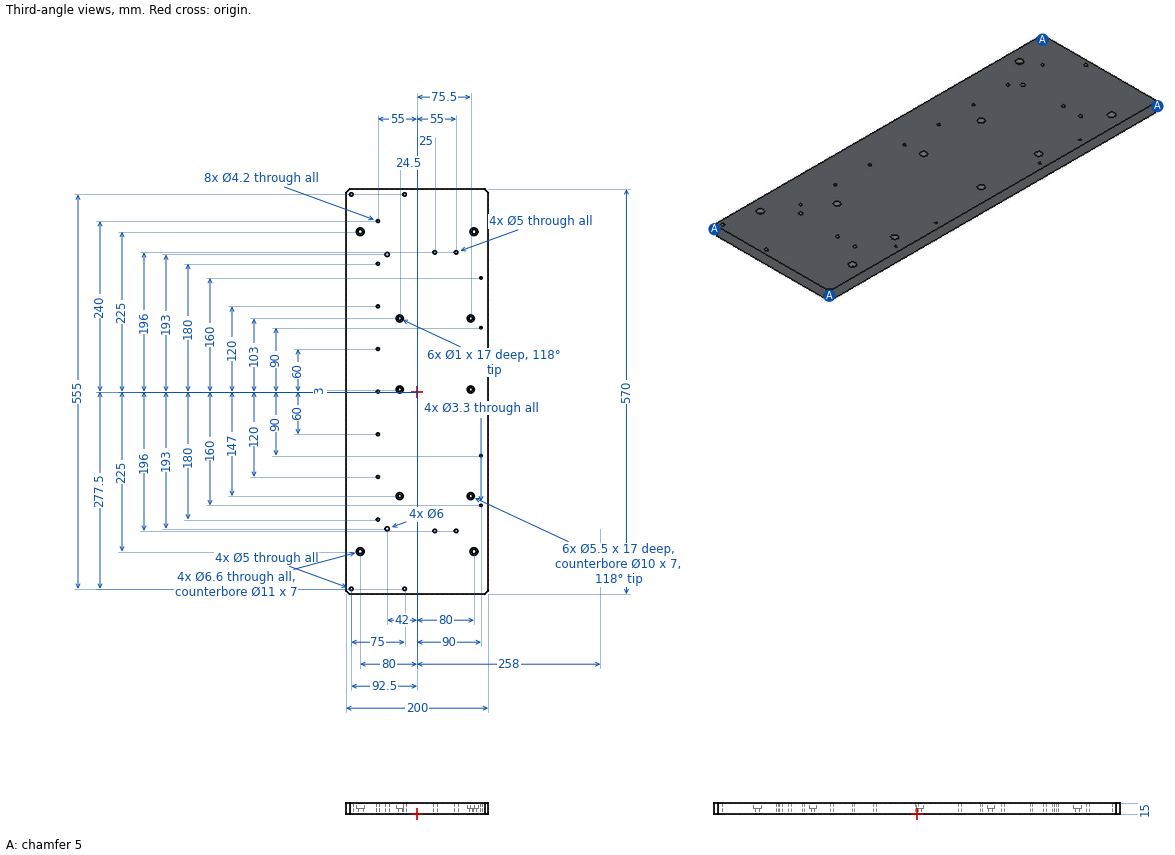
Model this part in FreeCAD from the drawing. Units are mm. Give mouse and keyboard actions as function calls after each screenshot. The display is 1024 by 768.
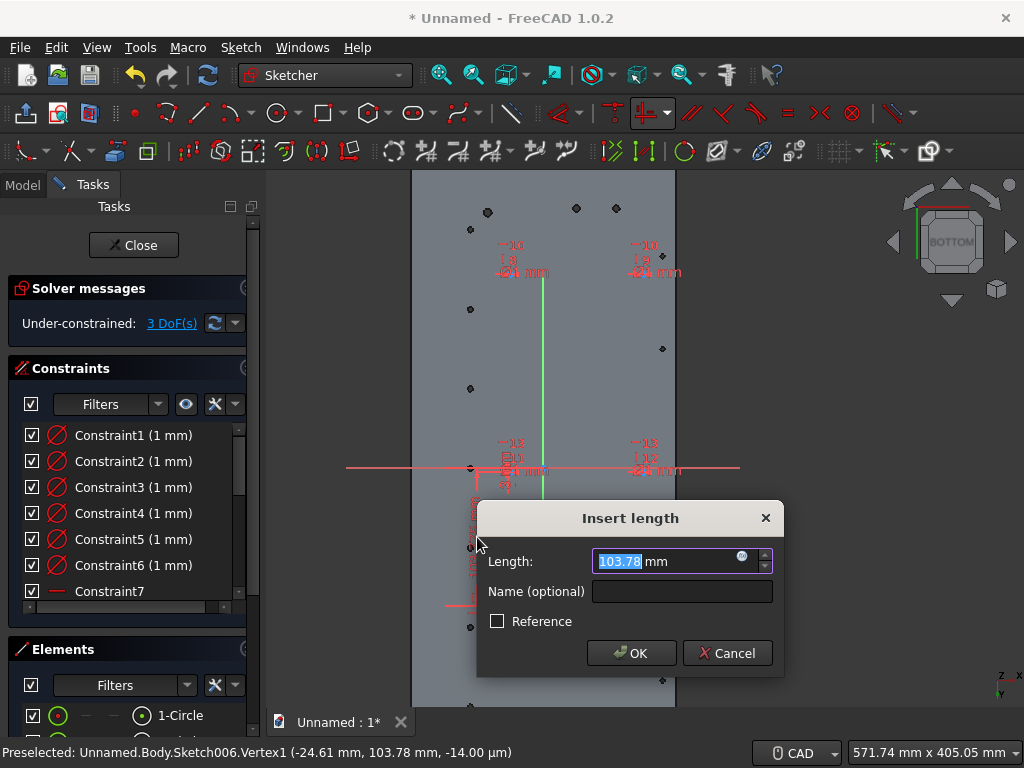
text(103)
key(Return)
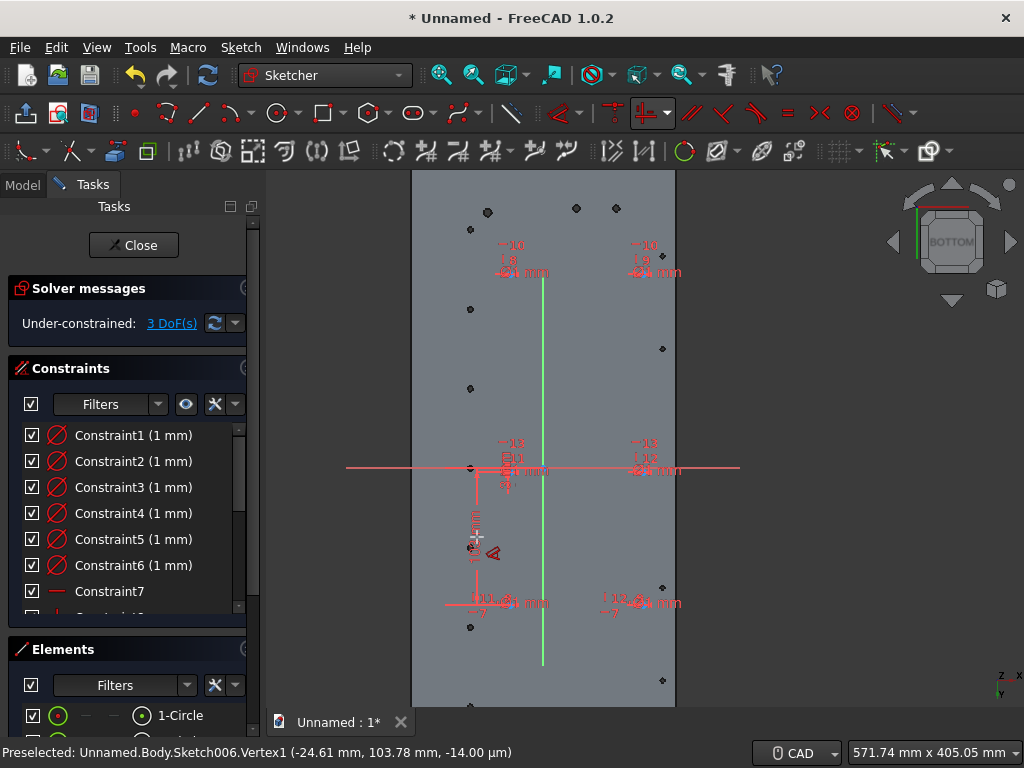
click(511, 274)
click(477, 371)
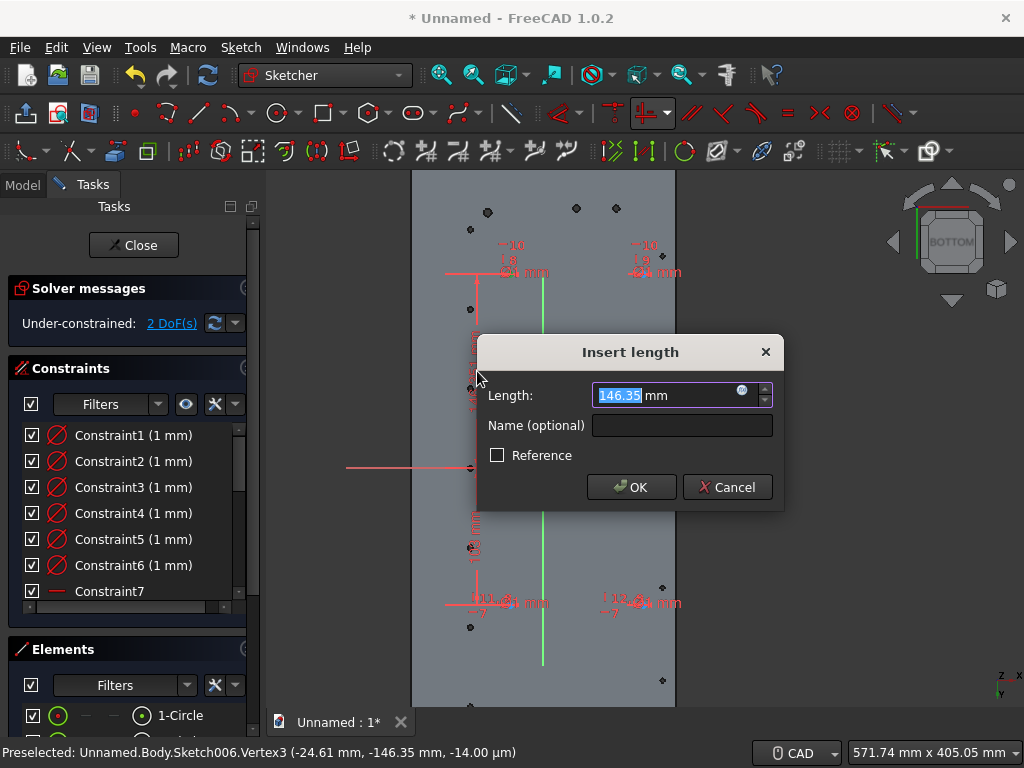
text(147)
key(Return)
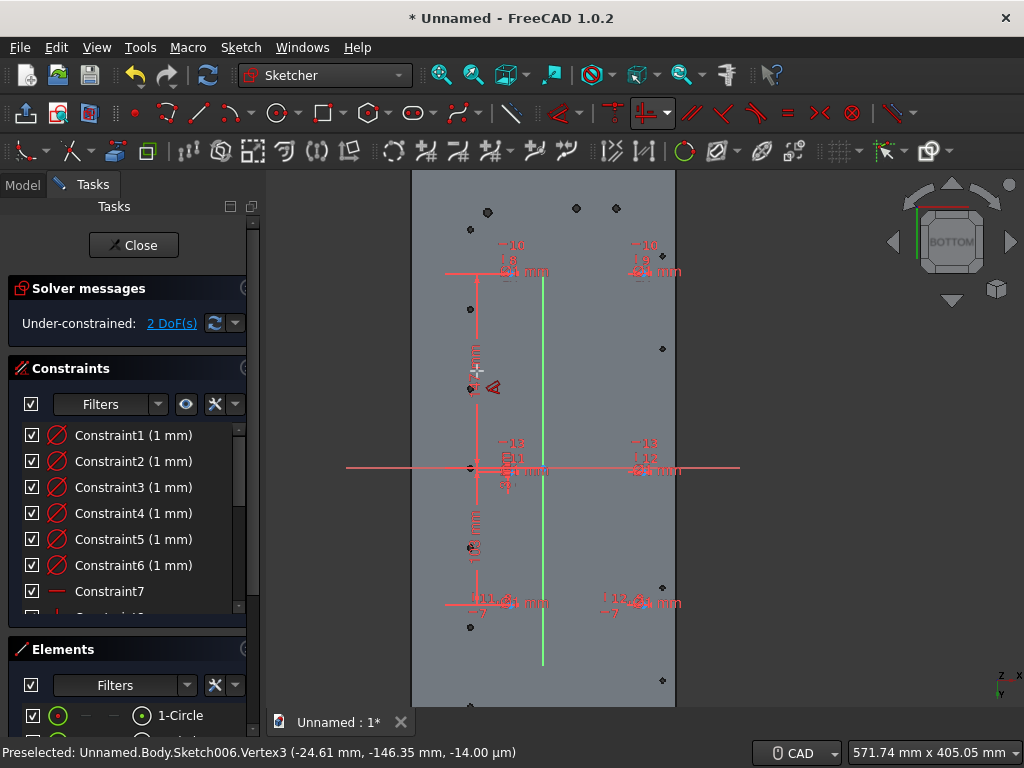
scroll(511, 605, up, 2)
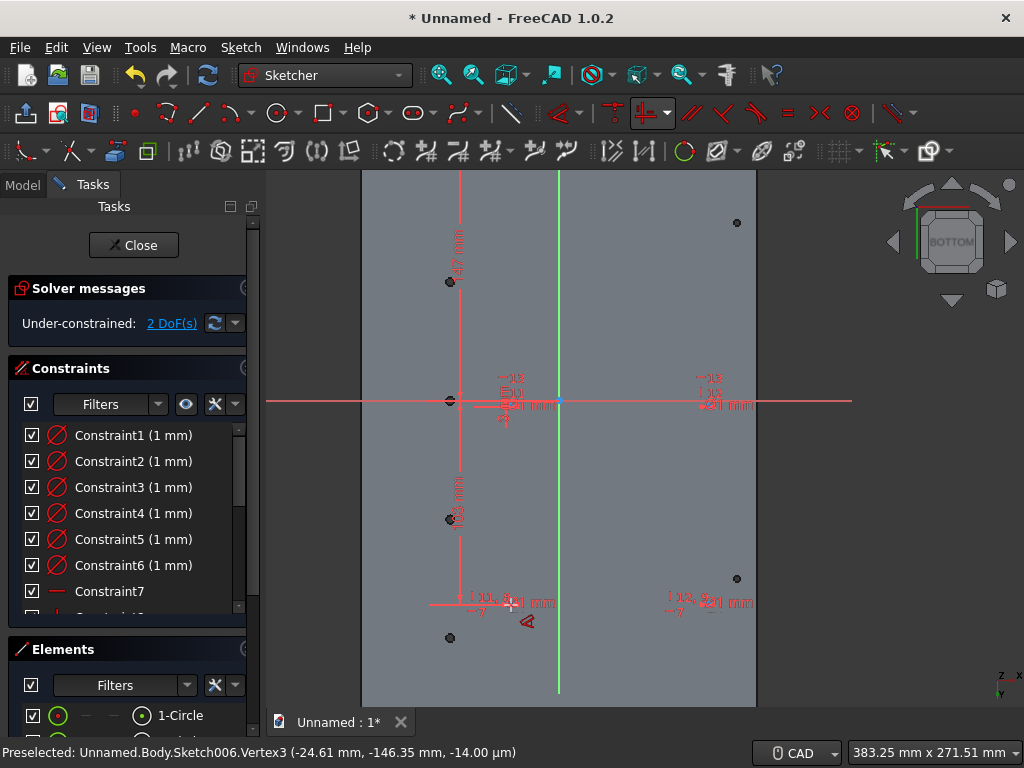
click(510, 605)
click(535, 639)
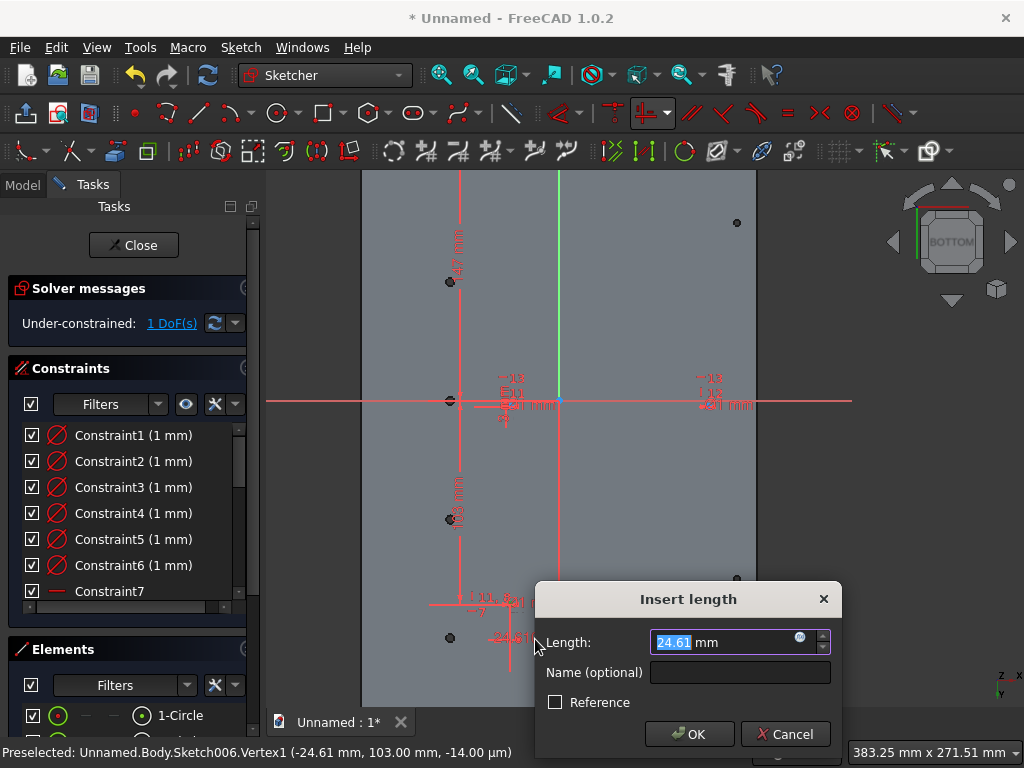
text(24.5)
key(Return)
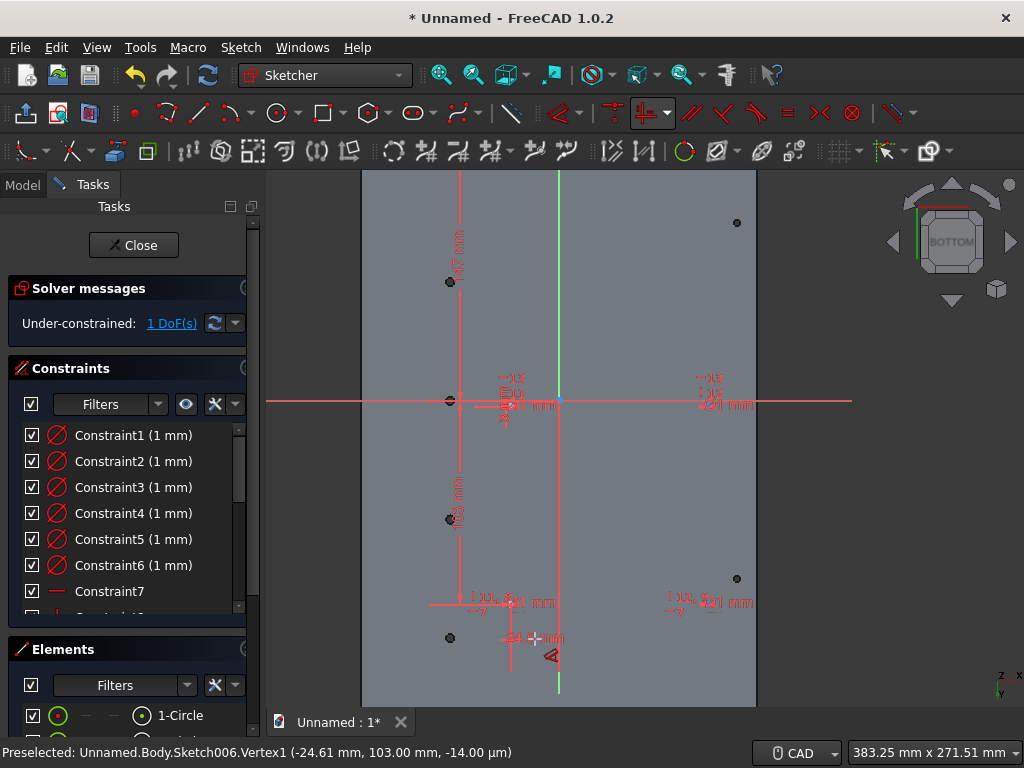
click(708, 605)
click(634, 639)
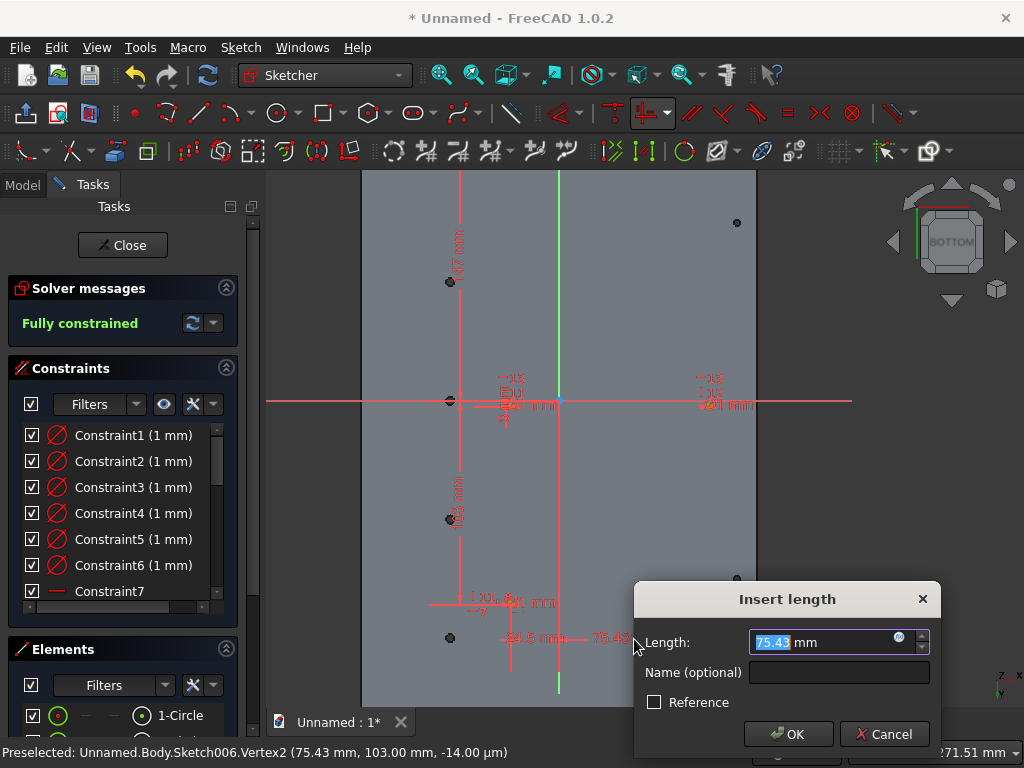
text(75.5)
key(Return)
key(Escape)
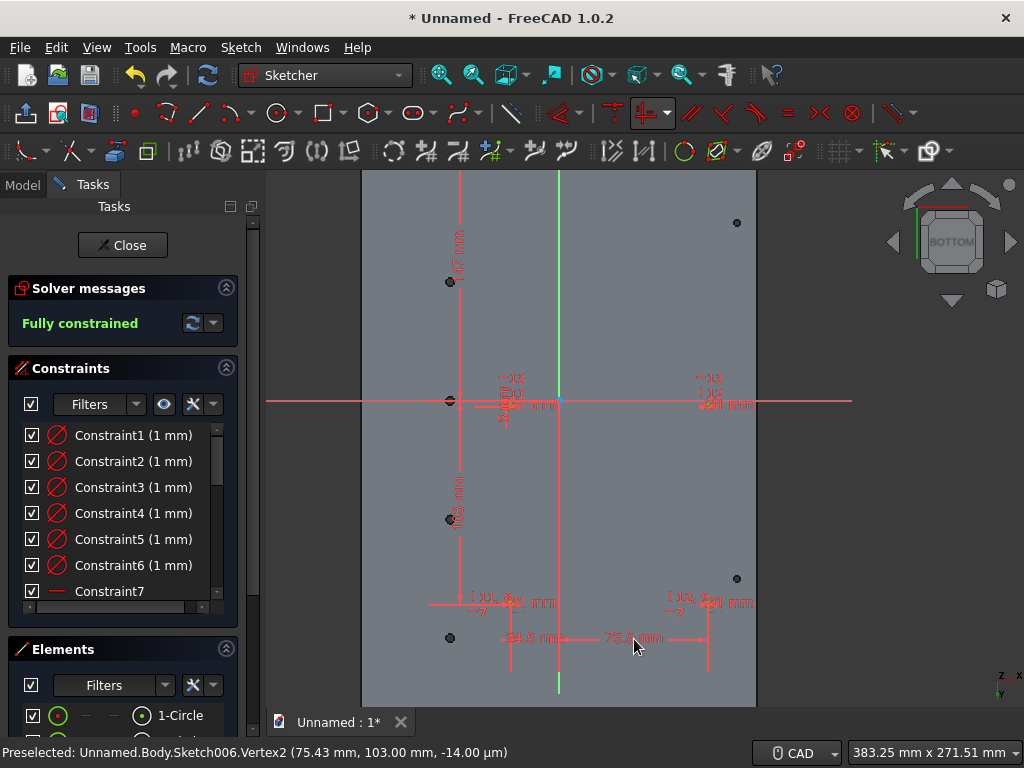
click(123, 245)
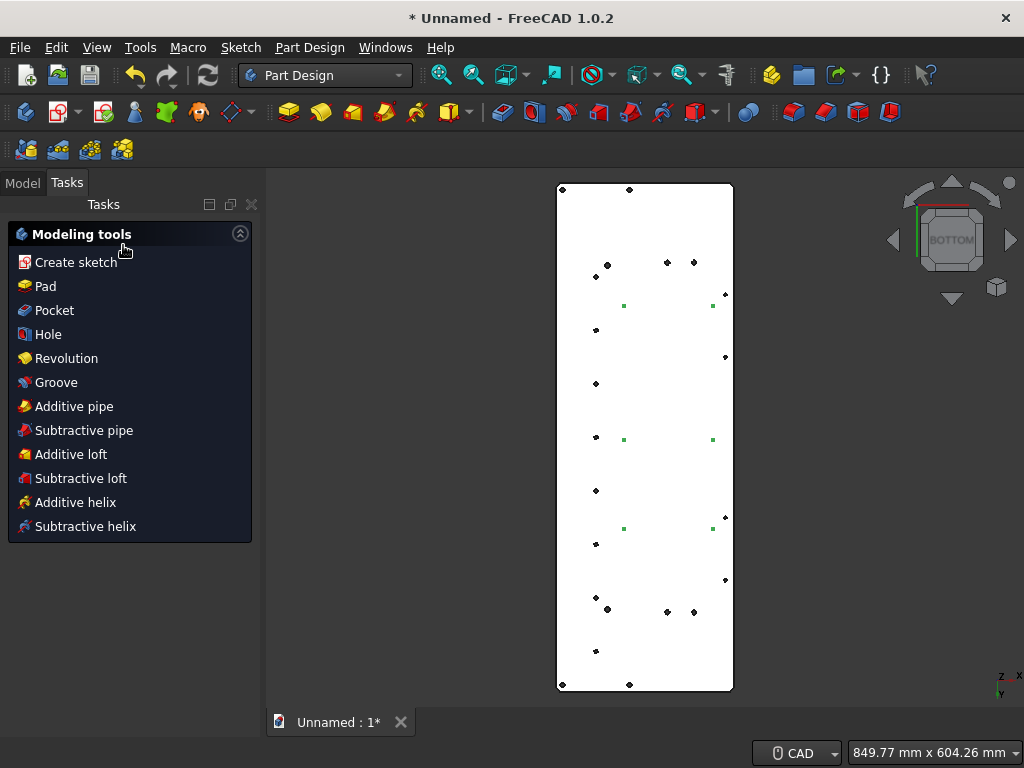
click(536, 112)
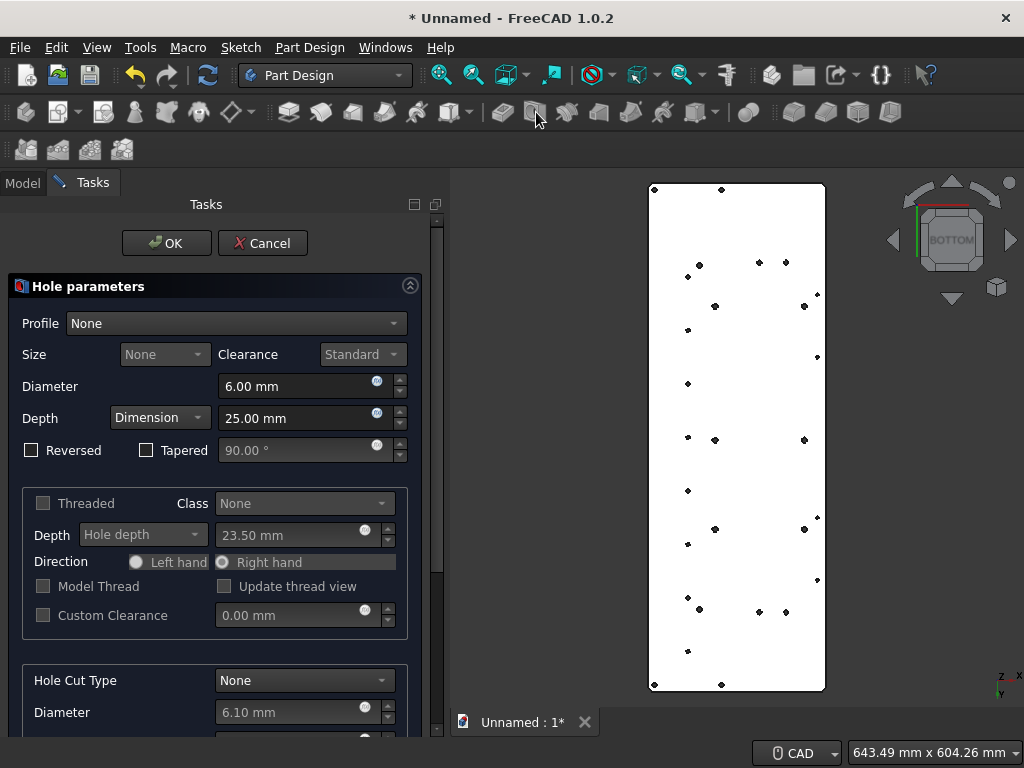
triple_click(305, 386)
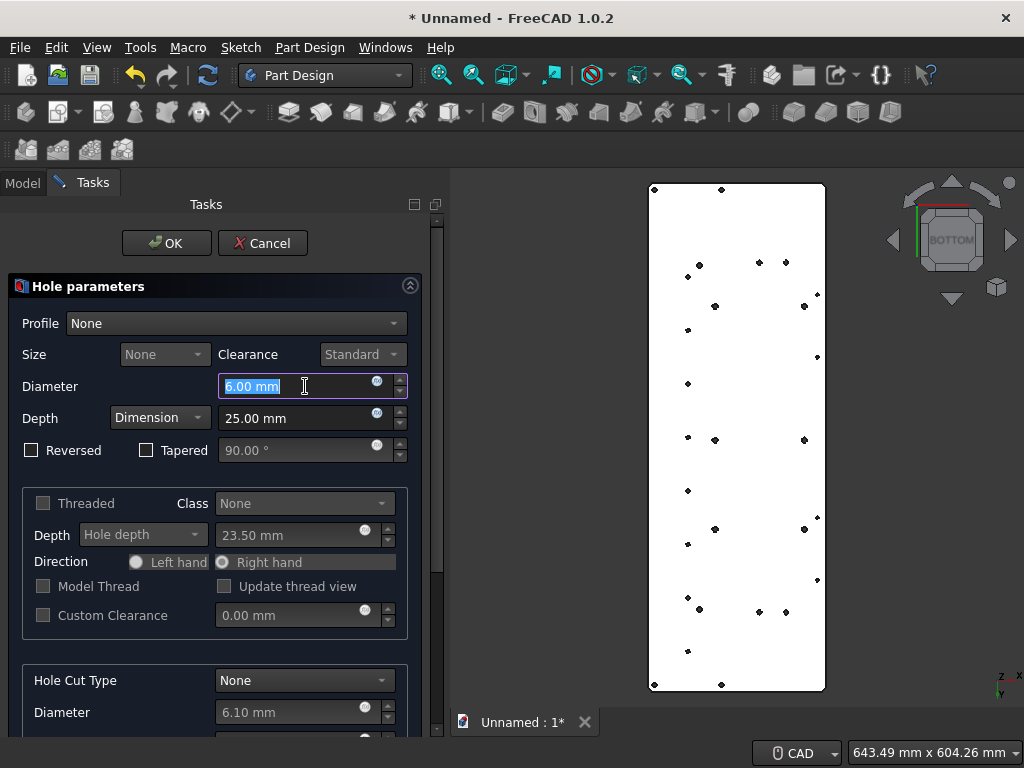
text(1)
key(Tab)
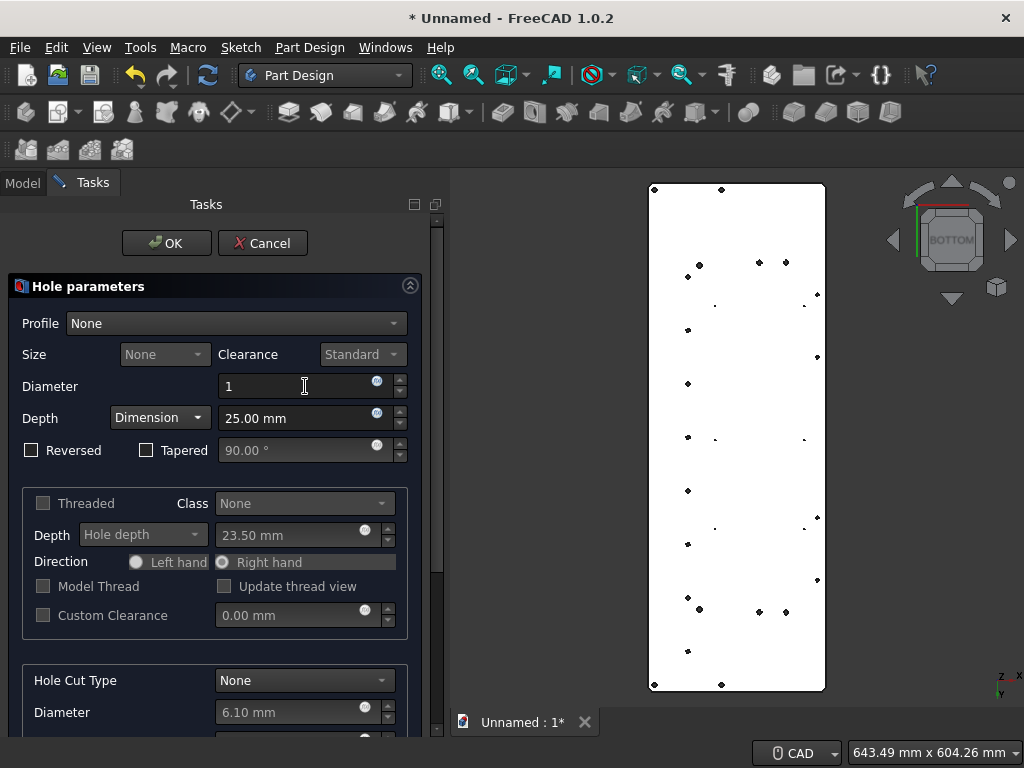
triple_click(305, 418)